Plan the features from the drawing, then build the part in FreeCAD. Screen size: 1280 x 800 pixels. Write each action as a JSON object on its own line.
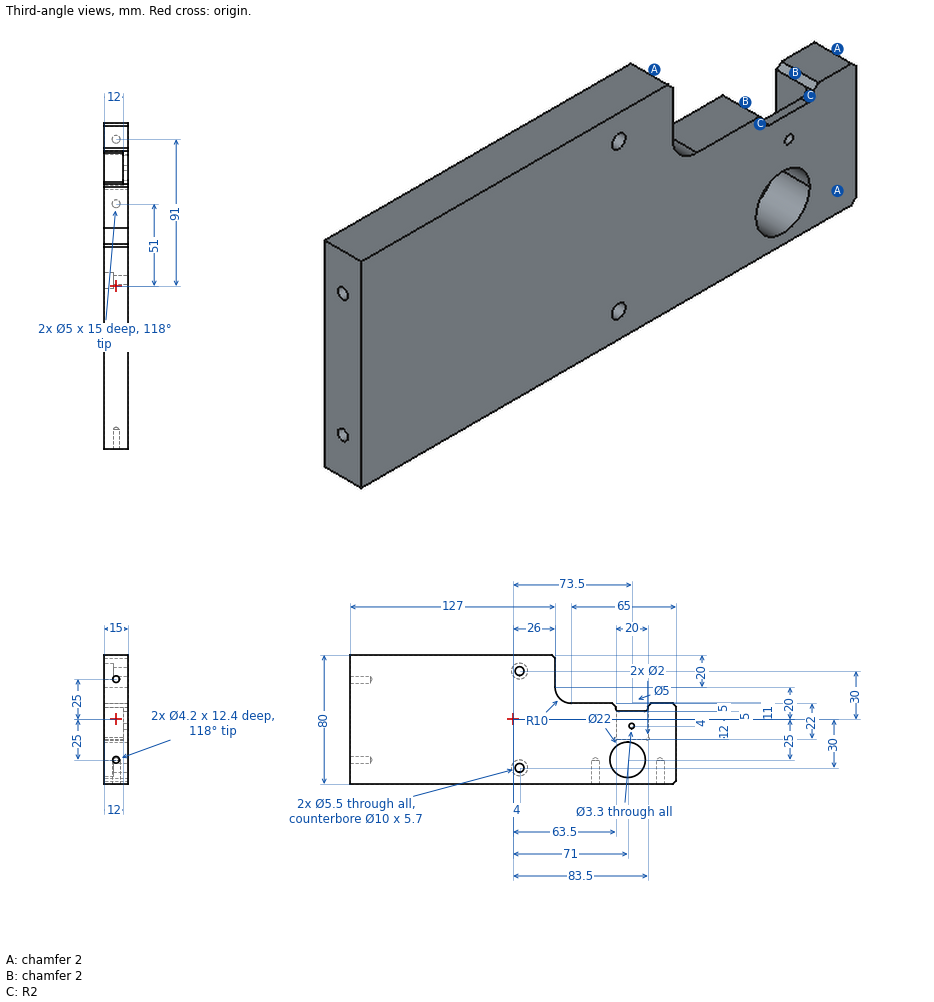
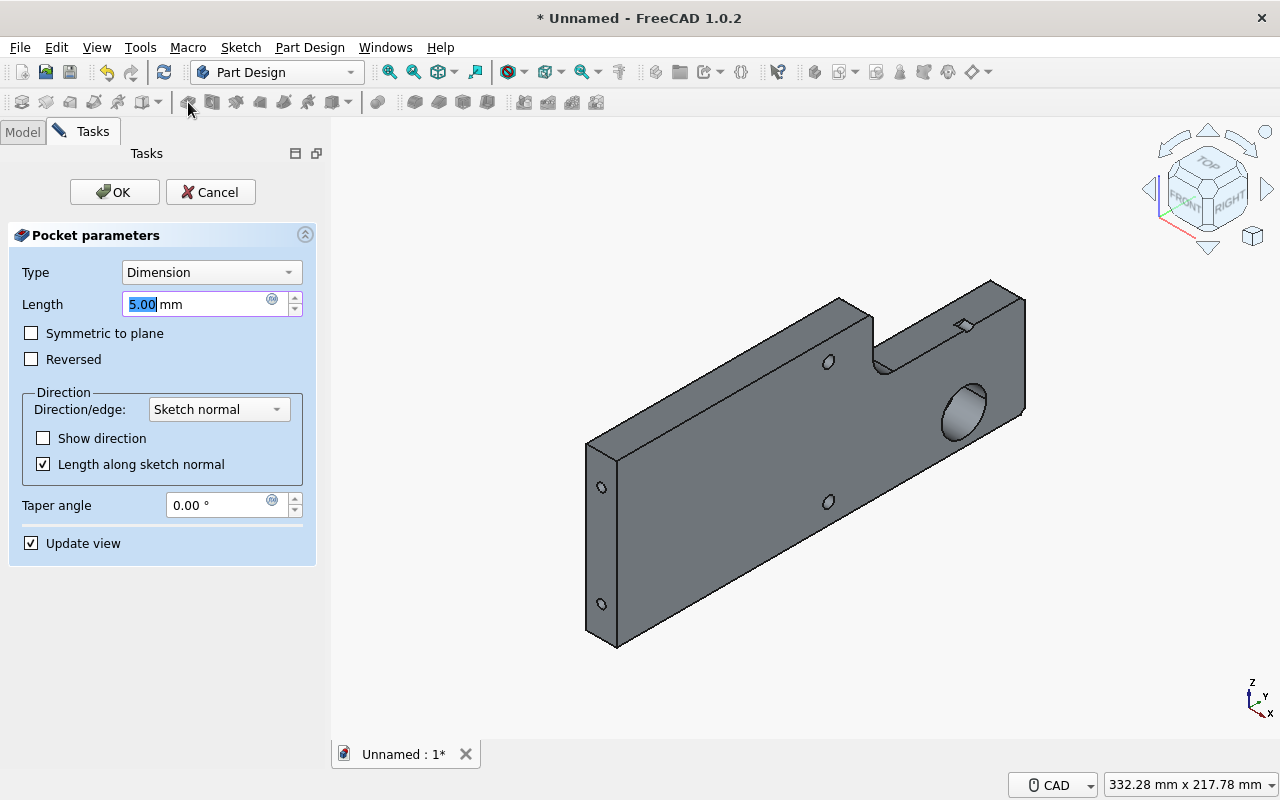
{"action": "left_click", "coordinate": [212, 272]}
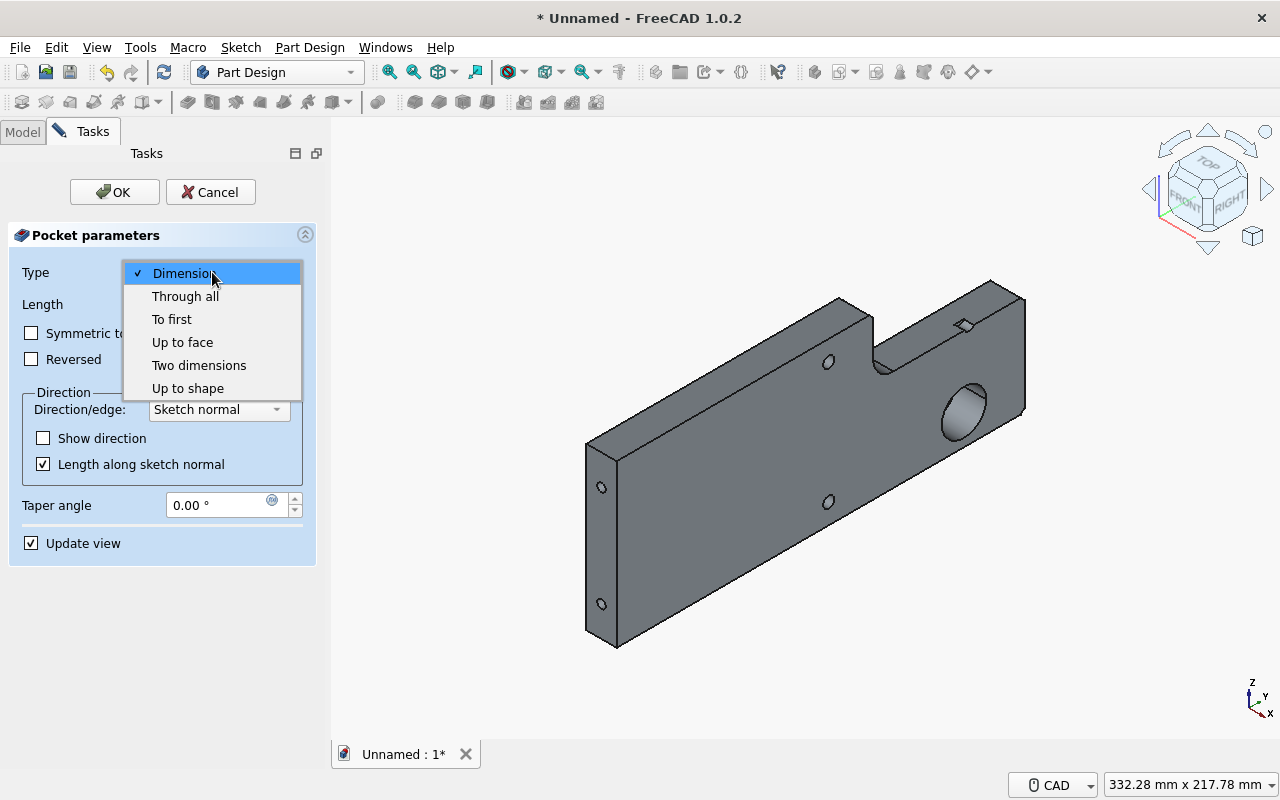
{"action": "left_click", "coordinate": [212, 296]}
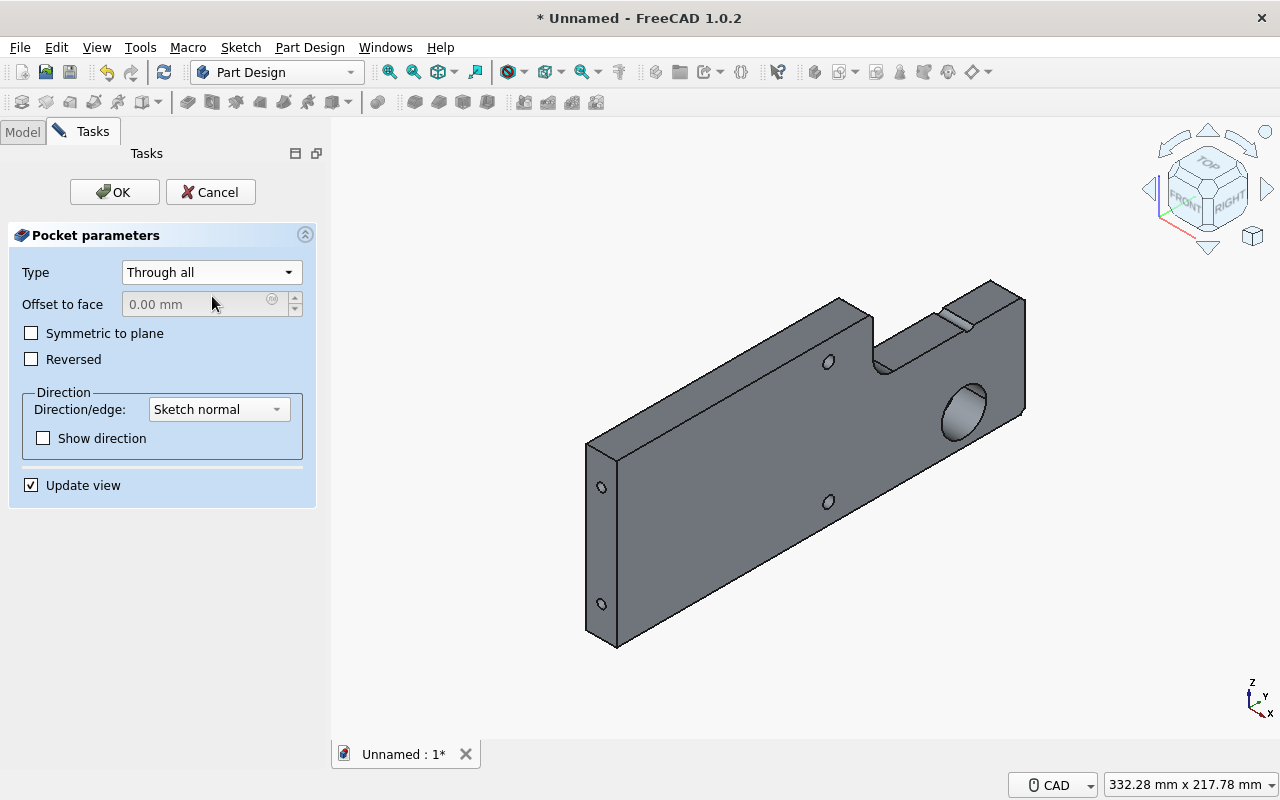
{"action": "left_click", "coordinate": [115, 192]}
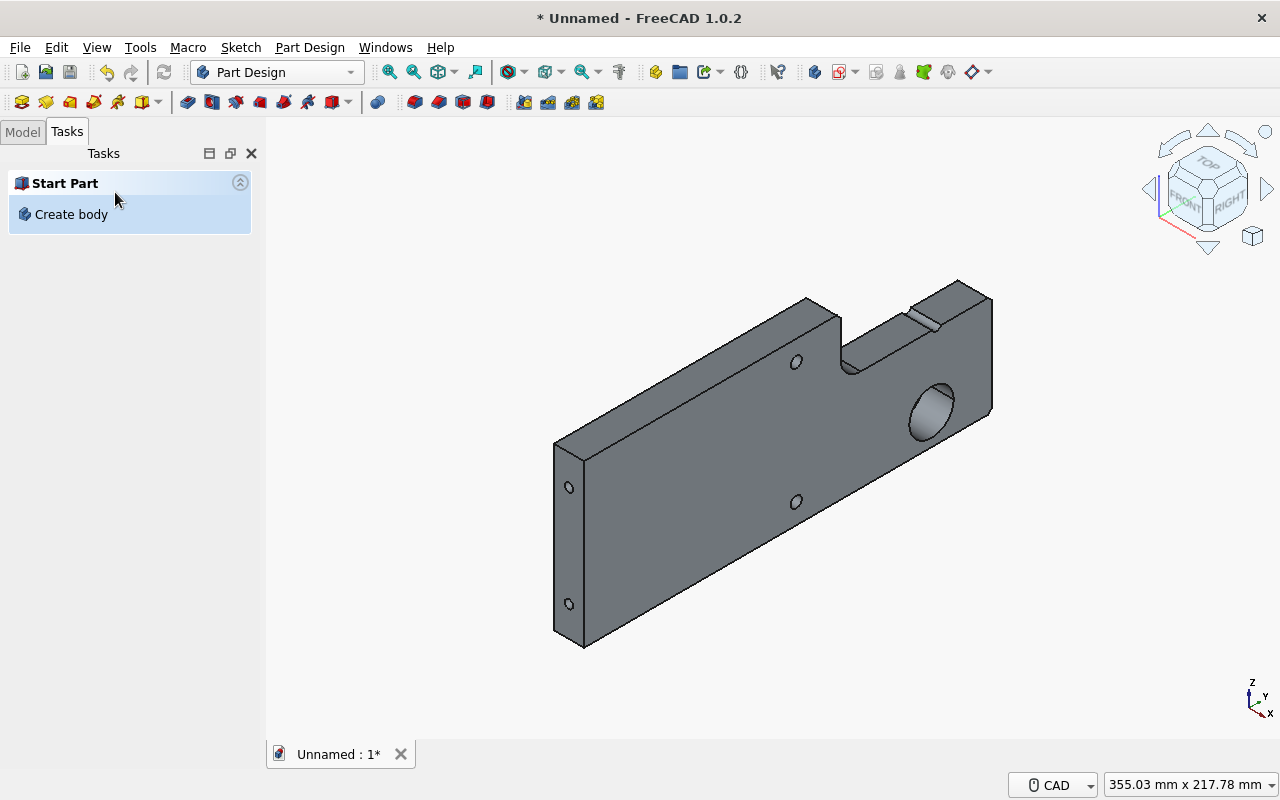
{"action": "key", "text": "6"}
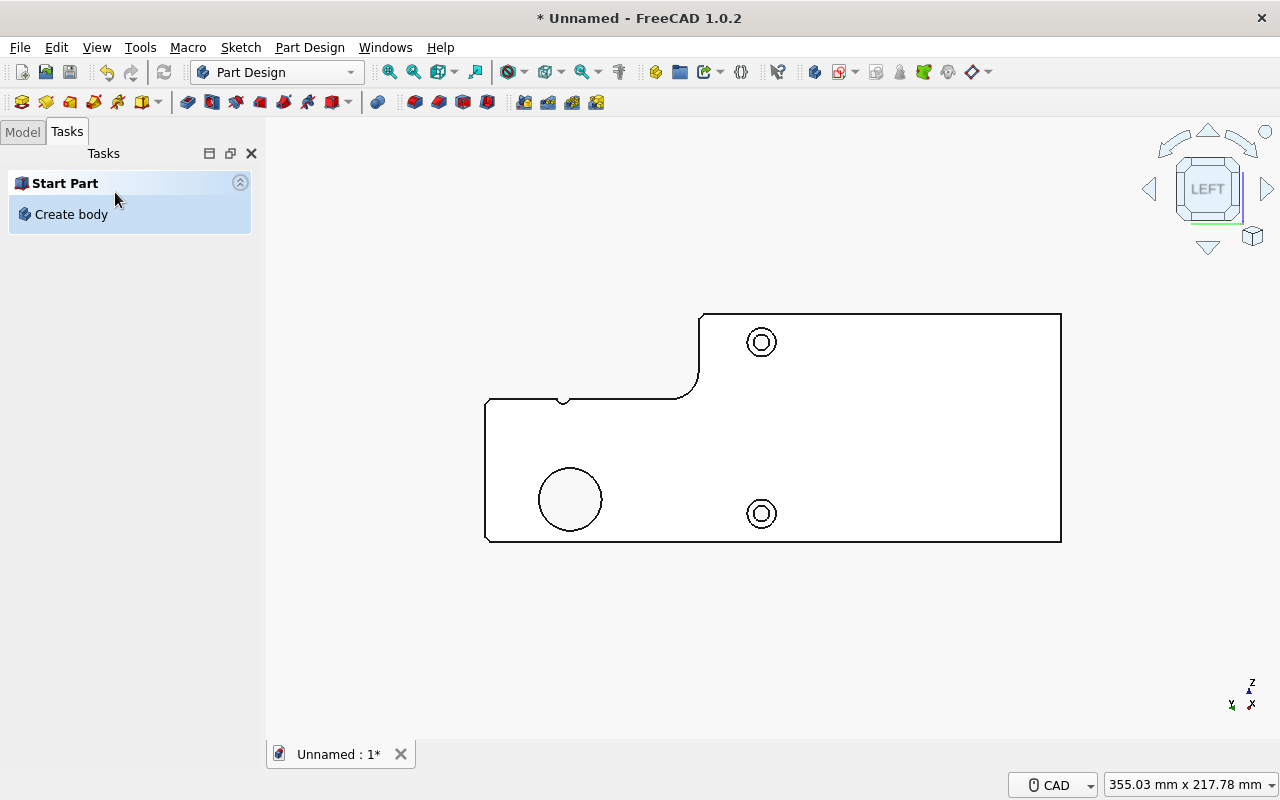
{"action": "left_click", "coordinate": [938, 427]}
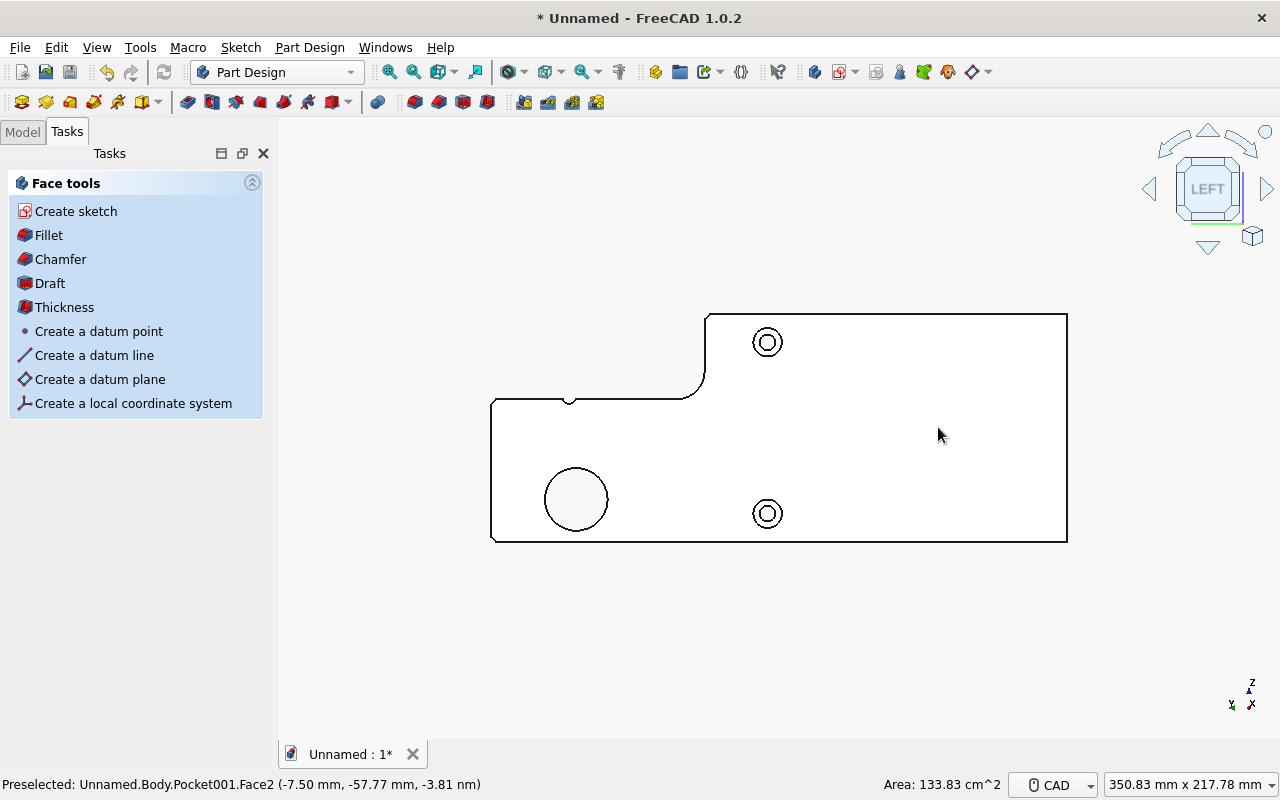
{"action": "left_click", "coordinate": [840, 72]}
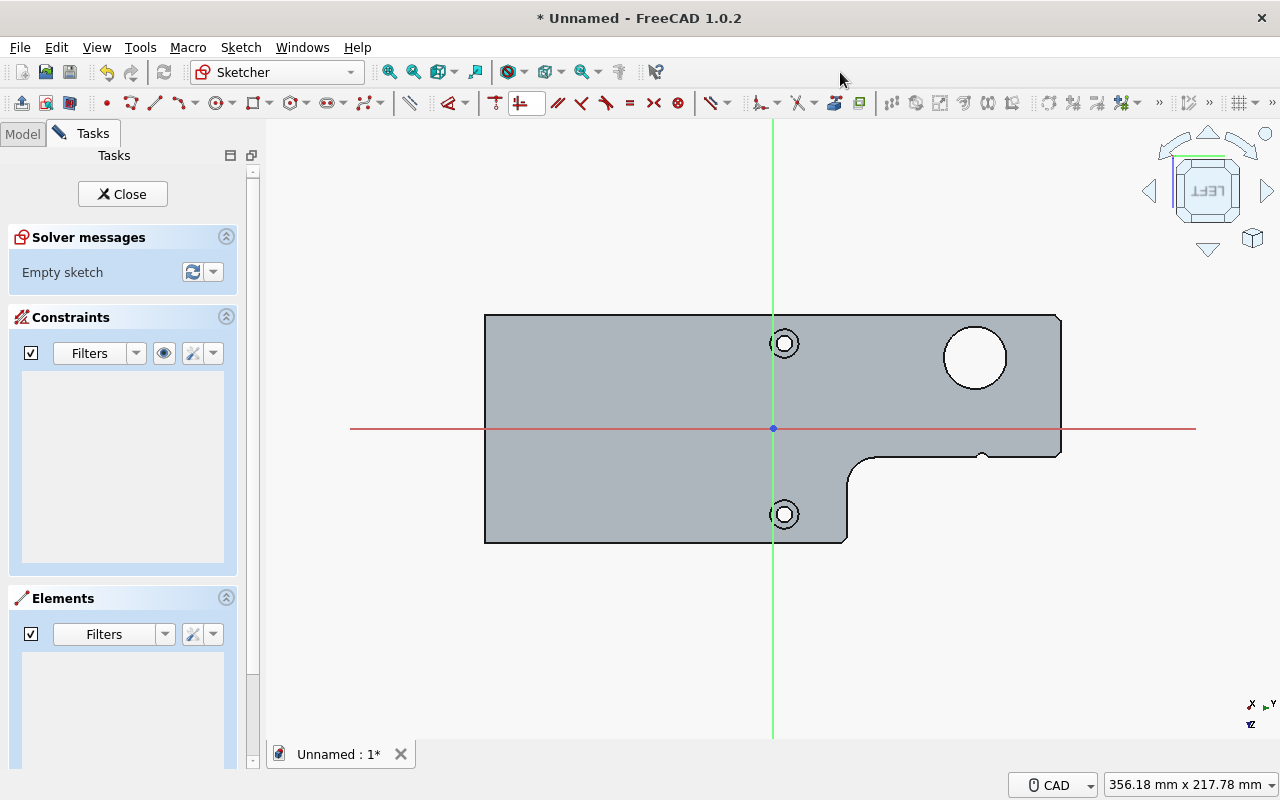
{"action": "scroll", "coordinate": [997, 417], "scroll_direction": "up", "scroll_amount": 15}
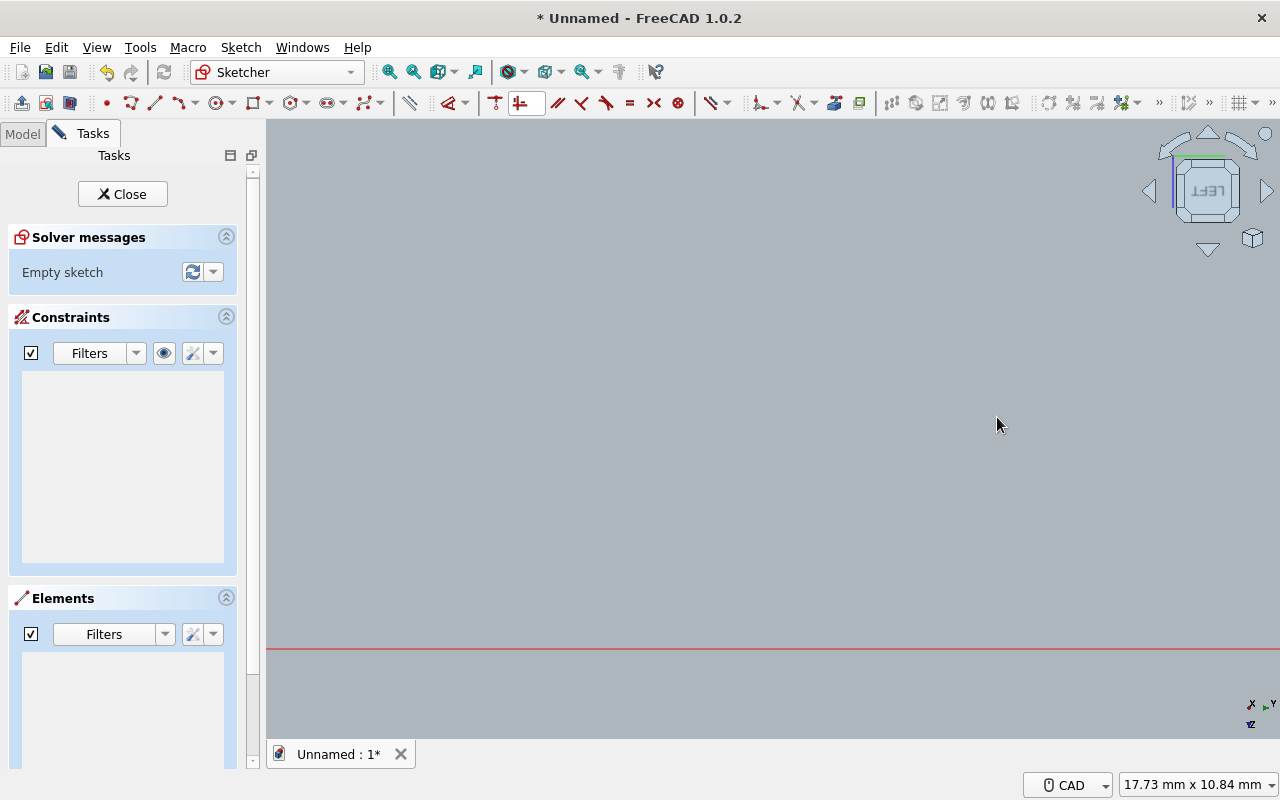
{"action": "scroll", "coordinate": [673, 413], "scroll_direction": "up", "scroll_amount": 4}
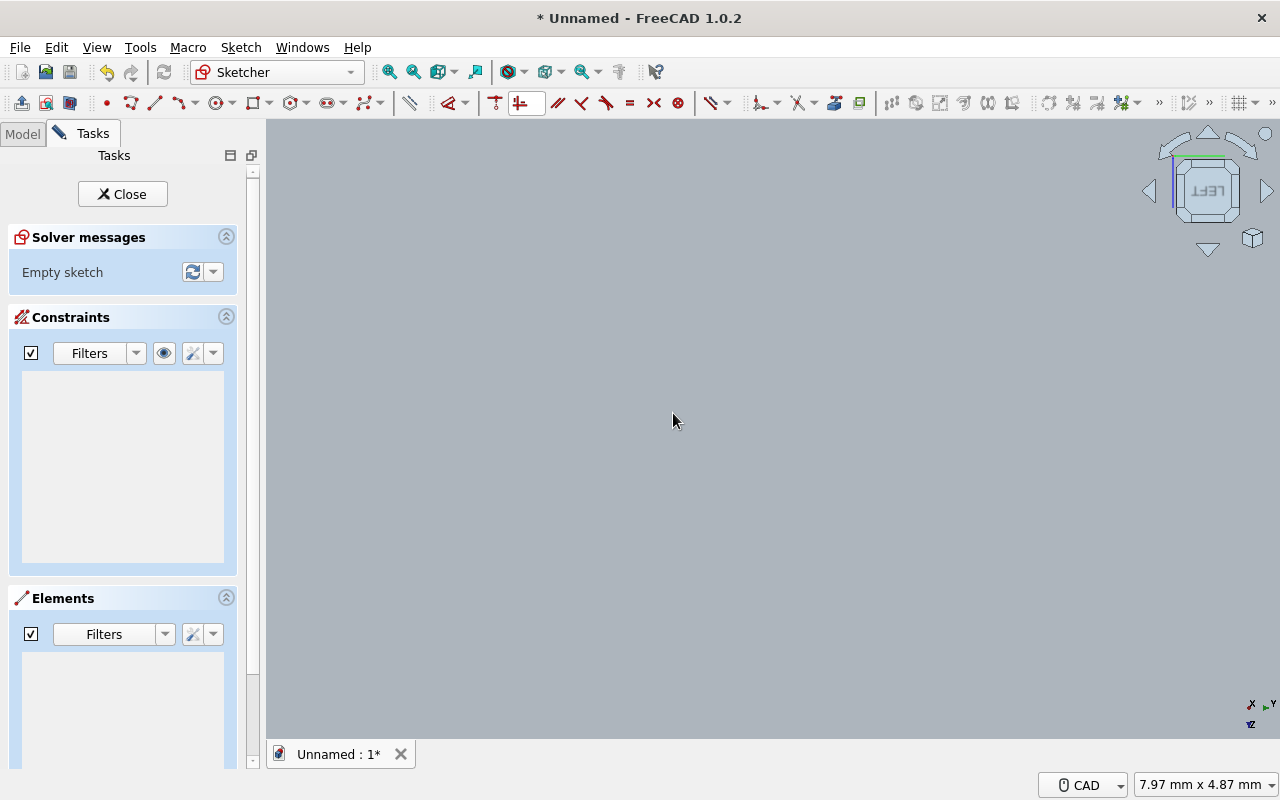
{"action": "left_click", "coordinate": [216, 104]}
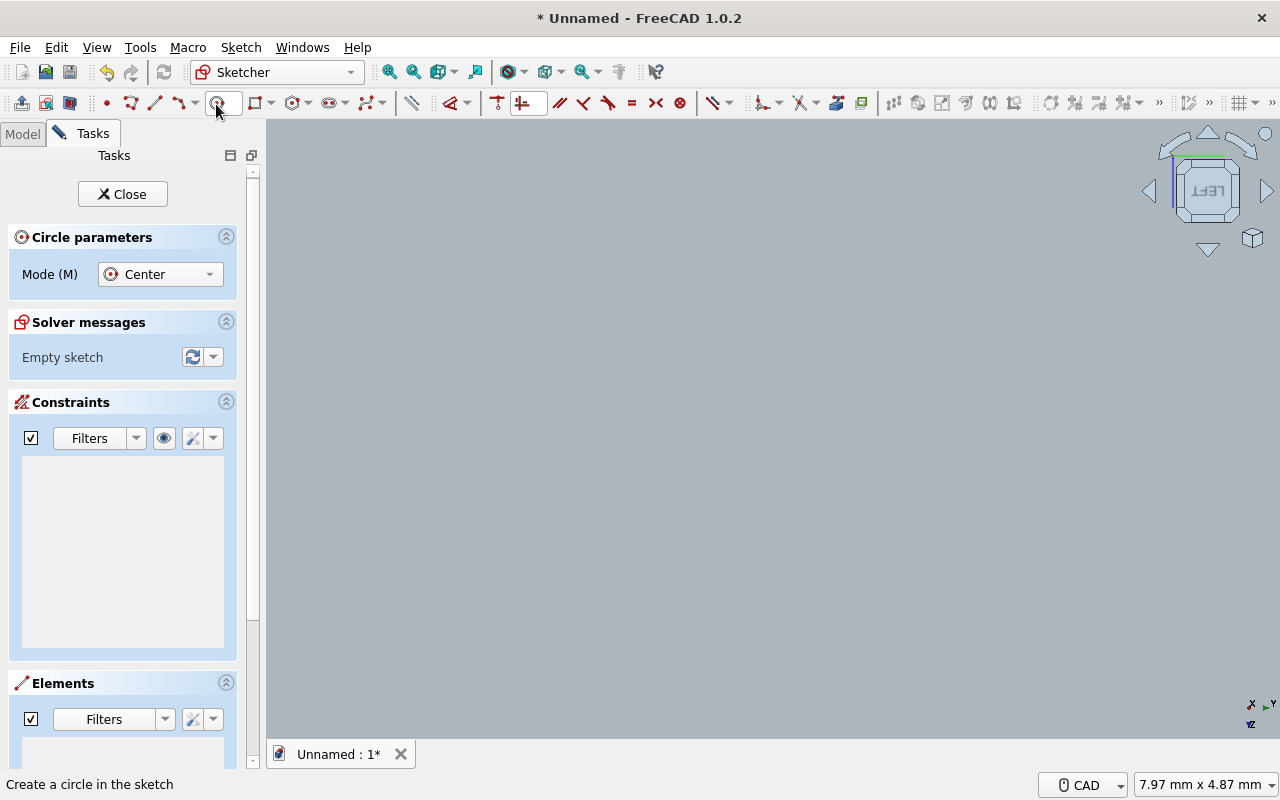
{"action": "left_click", "coordinate": [703, 428]}
{"action": "left_click", "coordinate": [852, 280]}
{"action": "key", "text": "Escape"}